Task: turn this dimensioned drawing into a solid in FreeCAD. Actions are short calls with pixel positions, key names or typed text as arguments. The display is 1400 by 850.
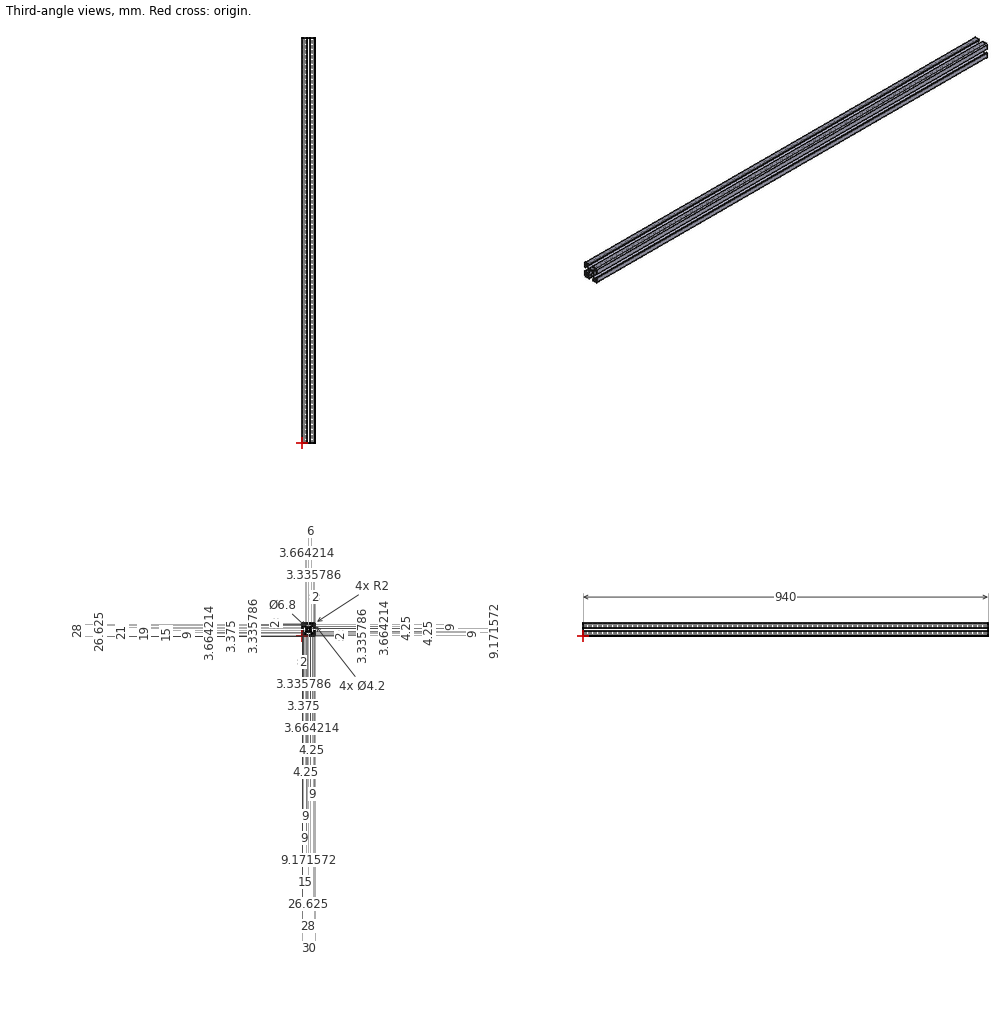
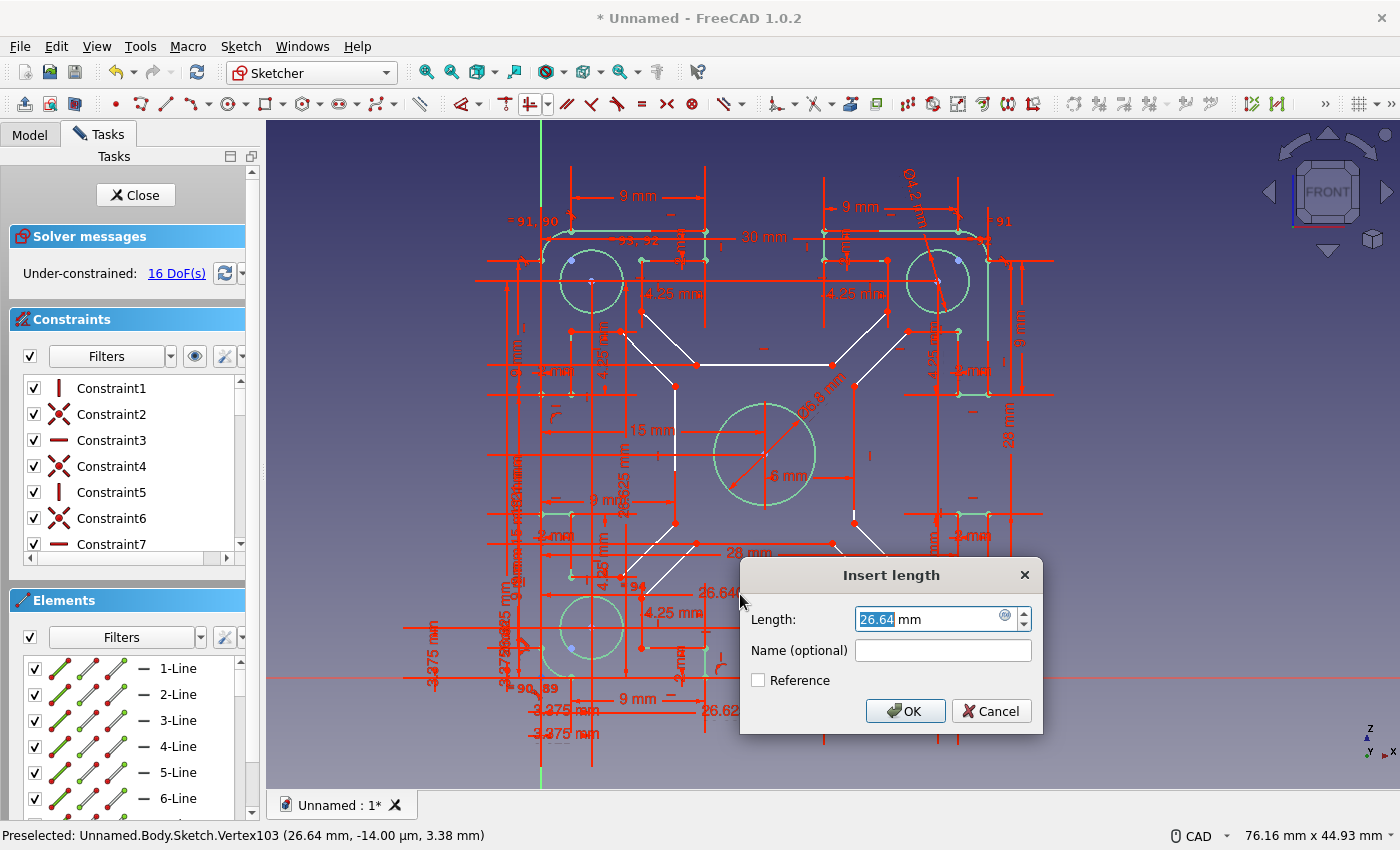
text(26.625)
key(Return)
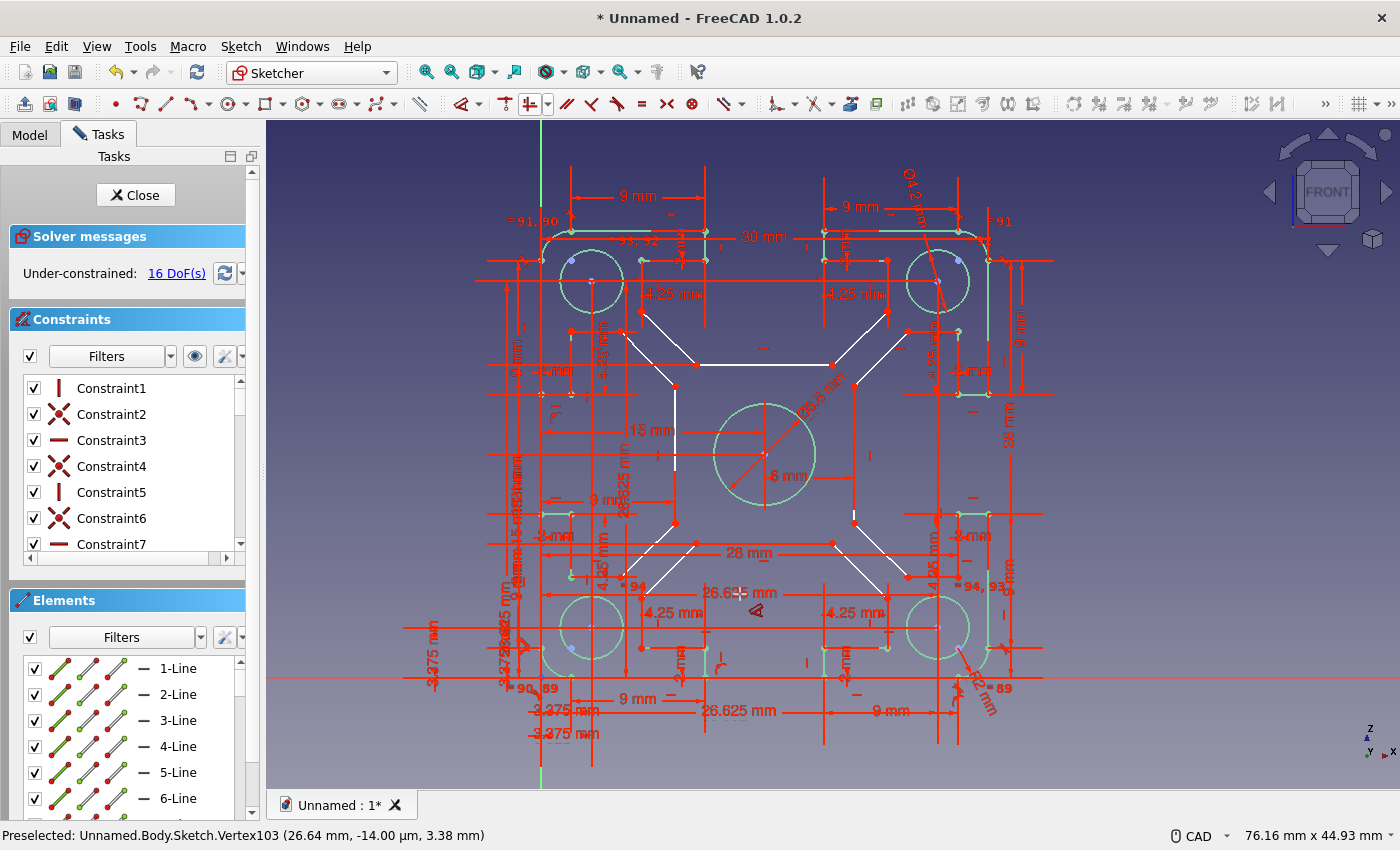
click(943, 332)
click(934, 298)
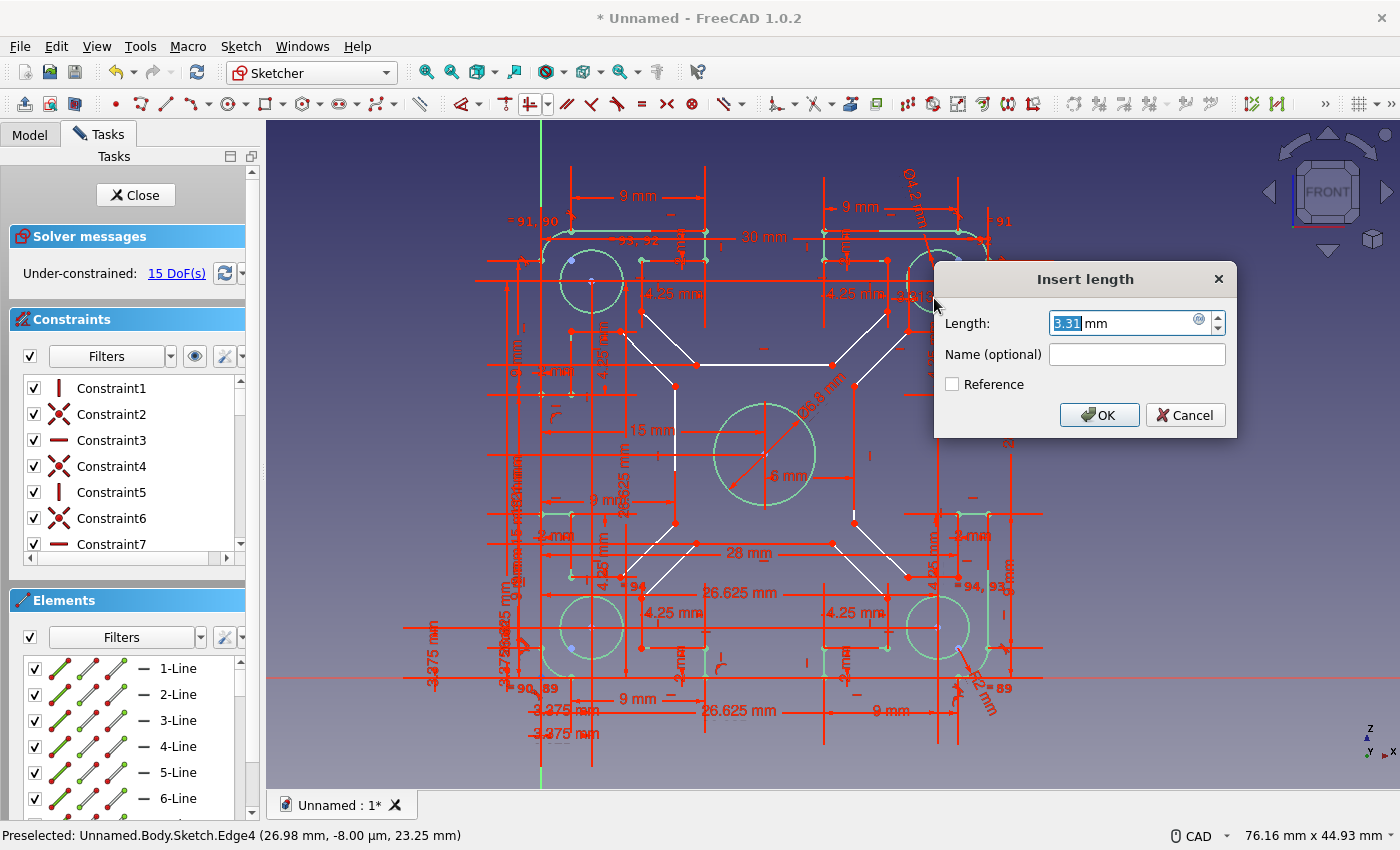
text(3.335786)
key(Return)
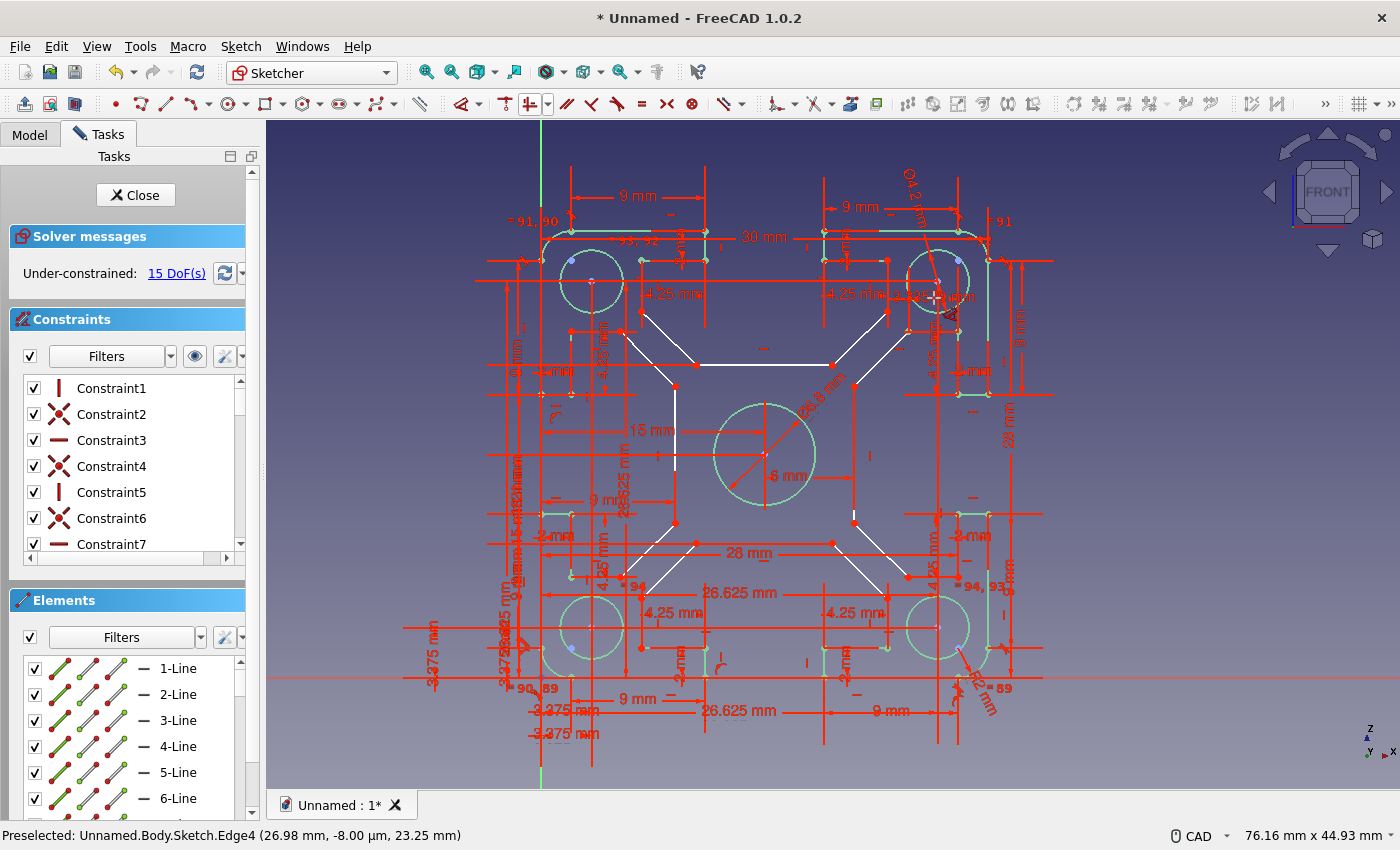
click(854, 428)
click(888, 455)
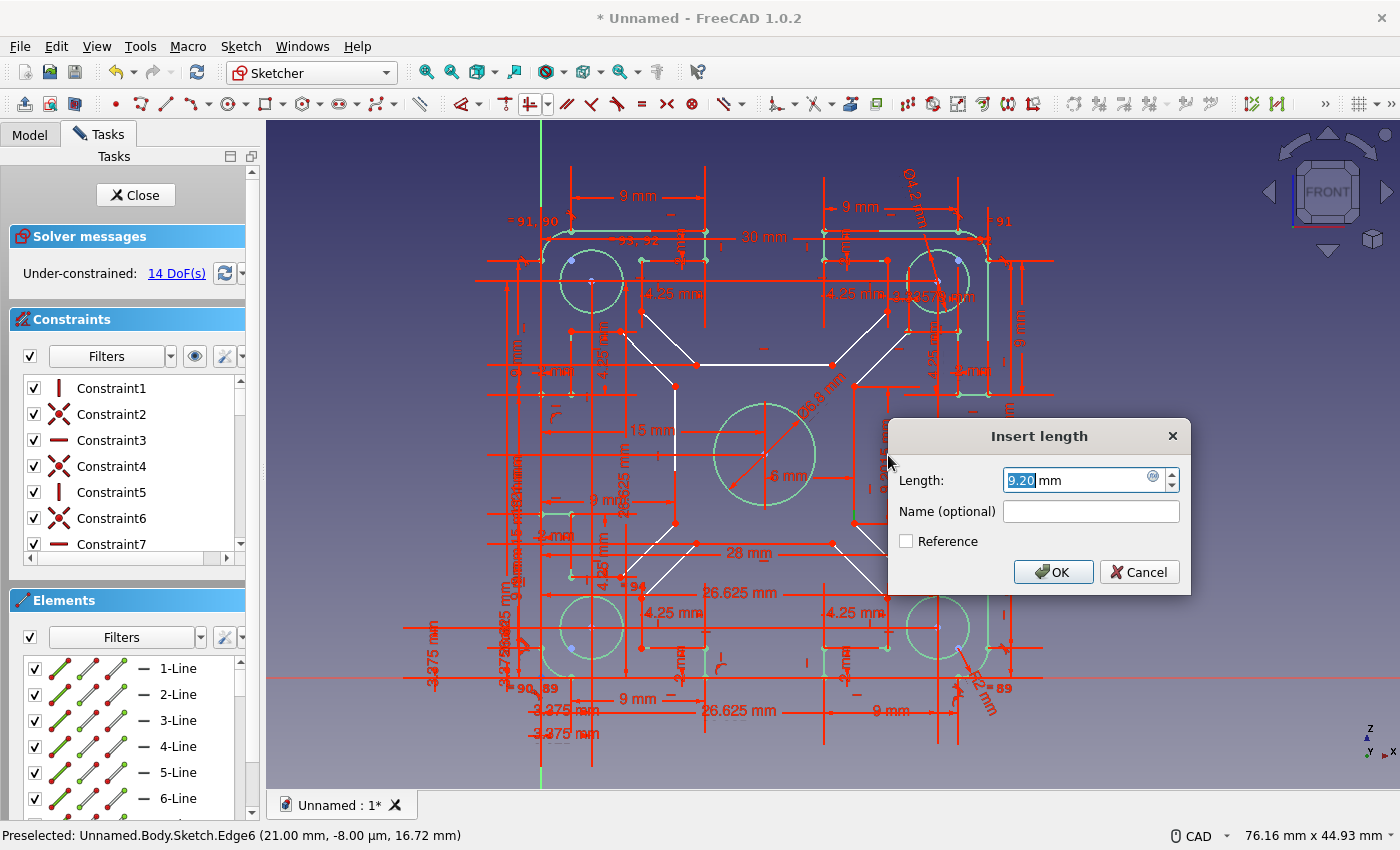
text(9.171572)
key(Return)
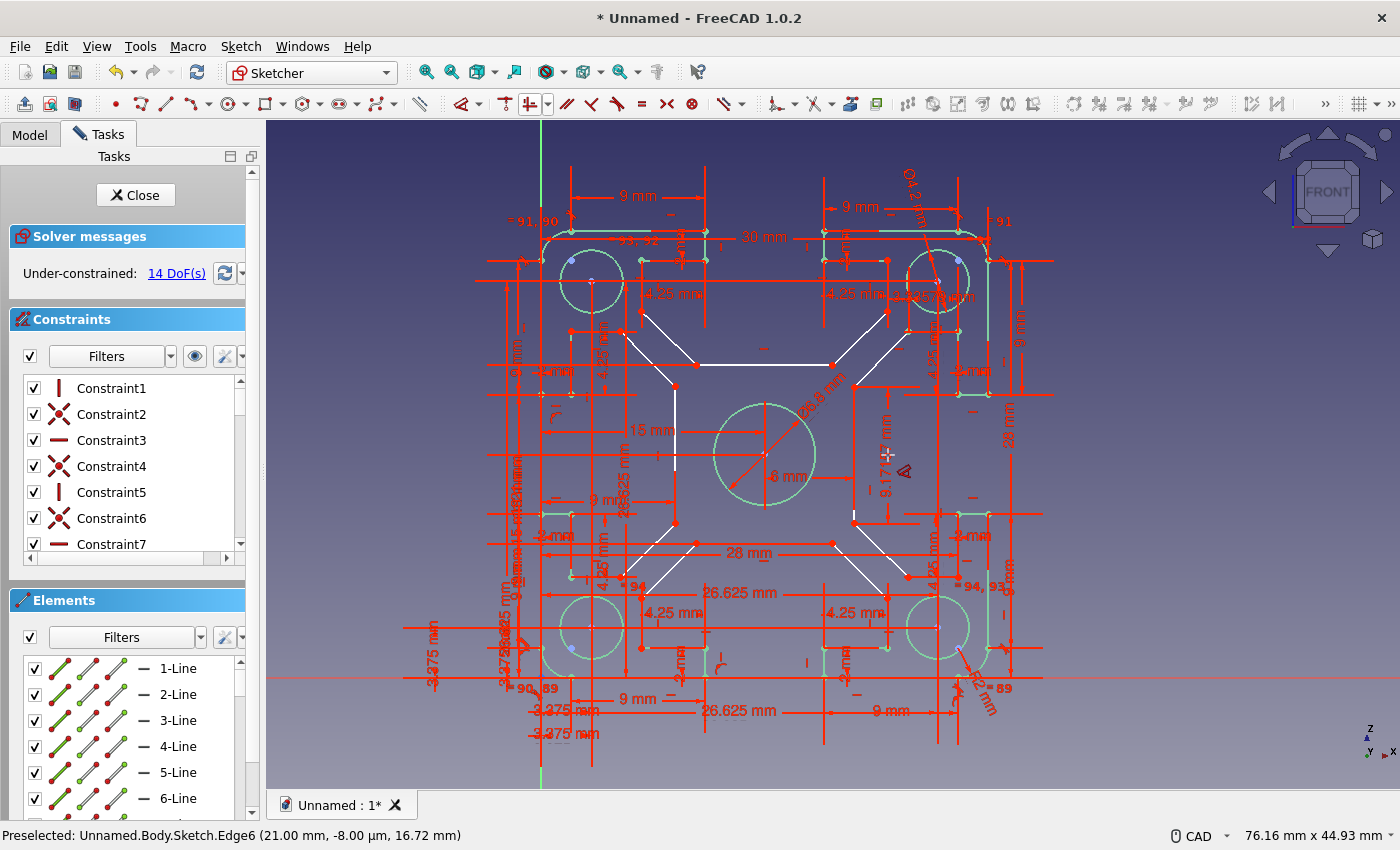
click(924, 577)
click(934, 611)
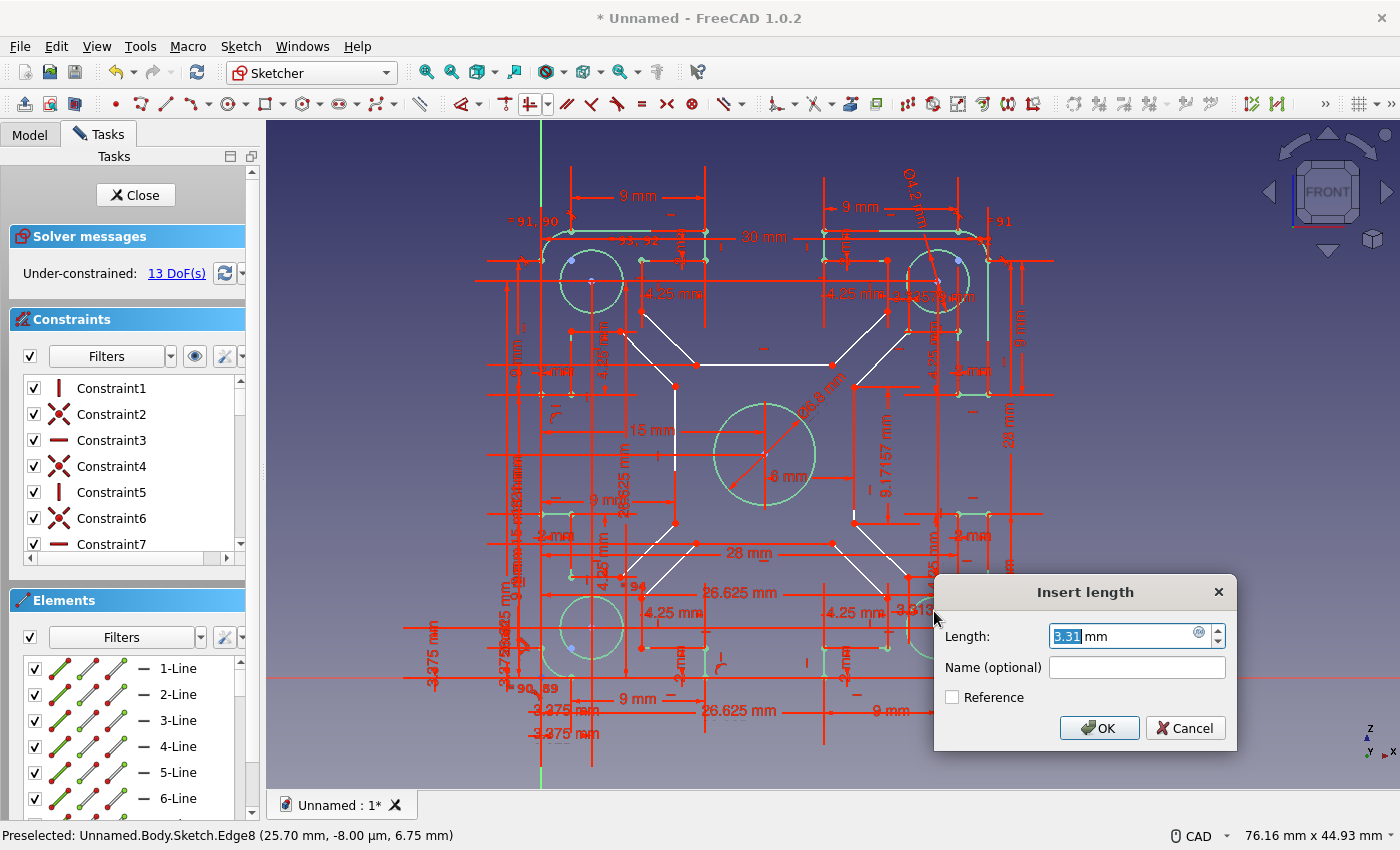
text(3.335786)
key(Return)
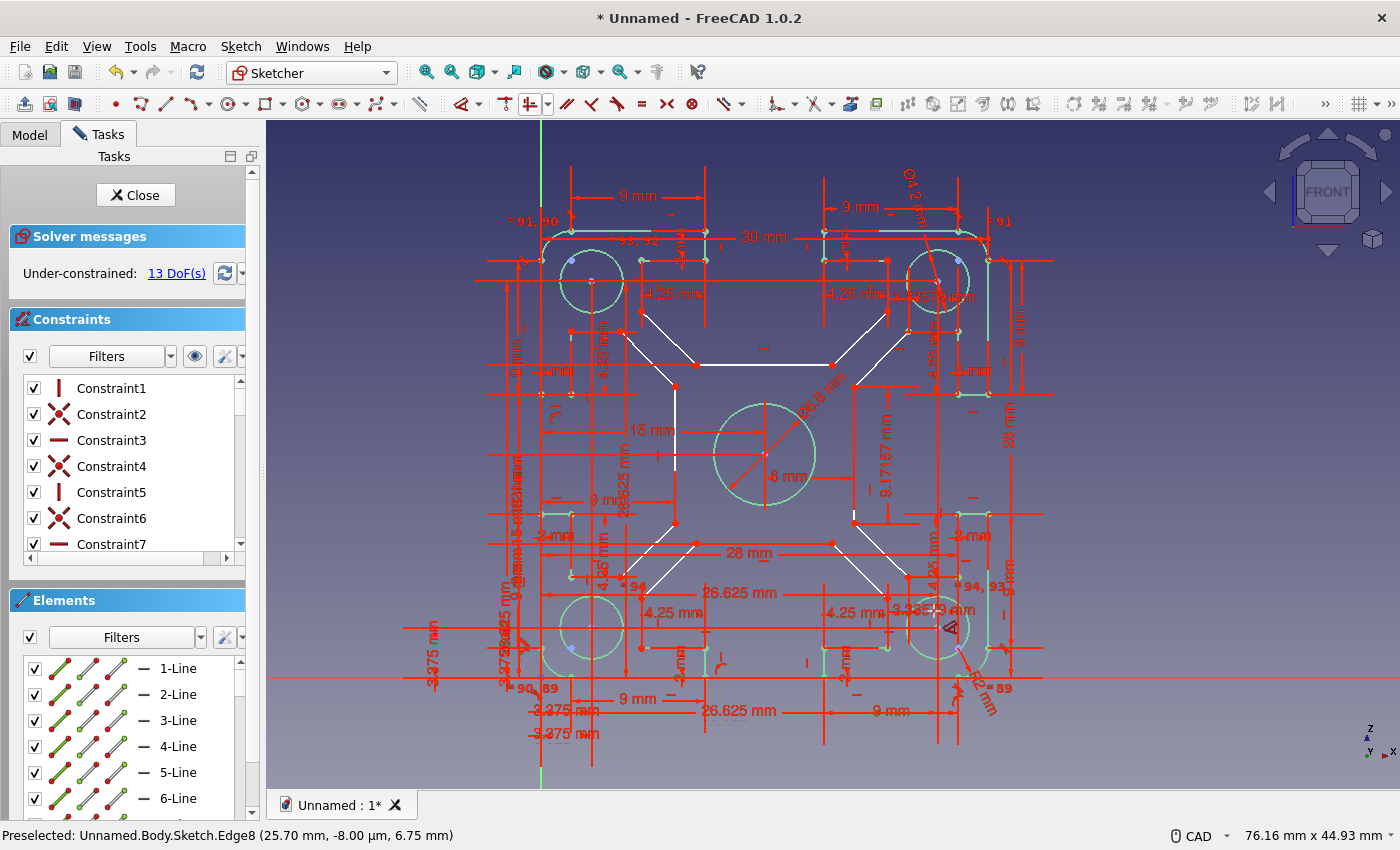
click(888, 633)
click(922, 635)